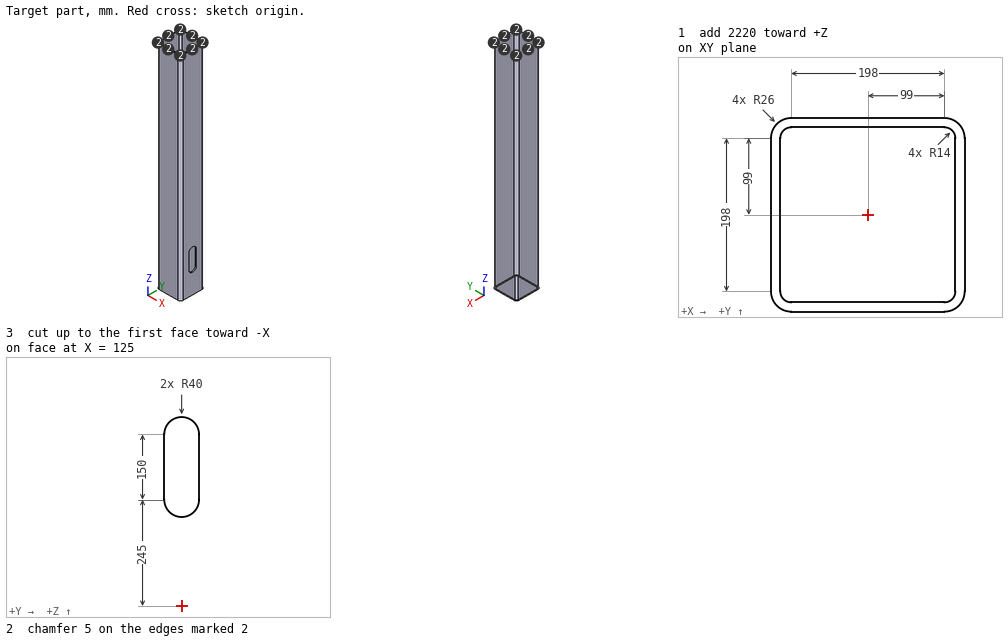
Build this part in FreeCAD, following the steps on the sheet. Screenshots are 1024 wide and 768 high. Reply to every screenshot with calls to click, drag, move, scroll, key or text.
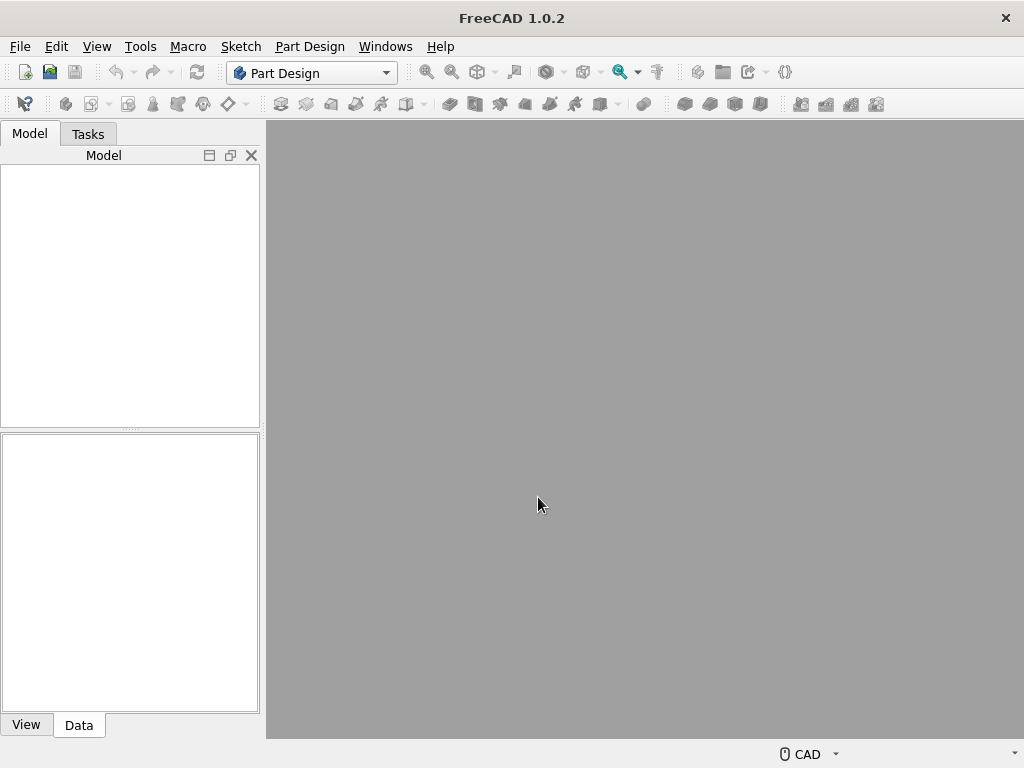
click(25, 72)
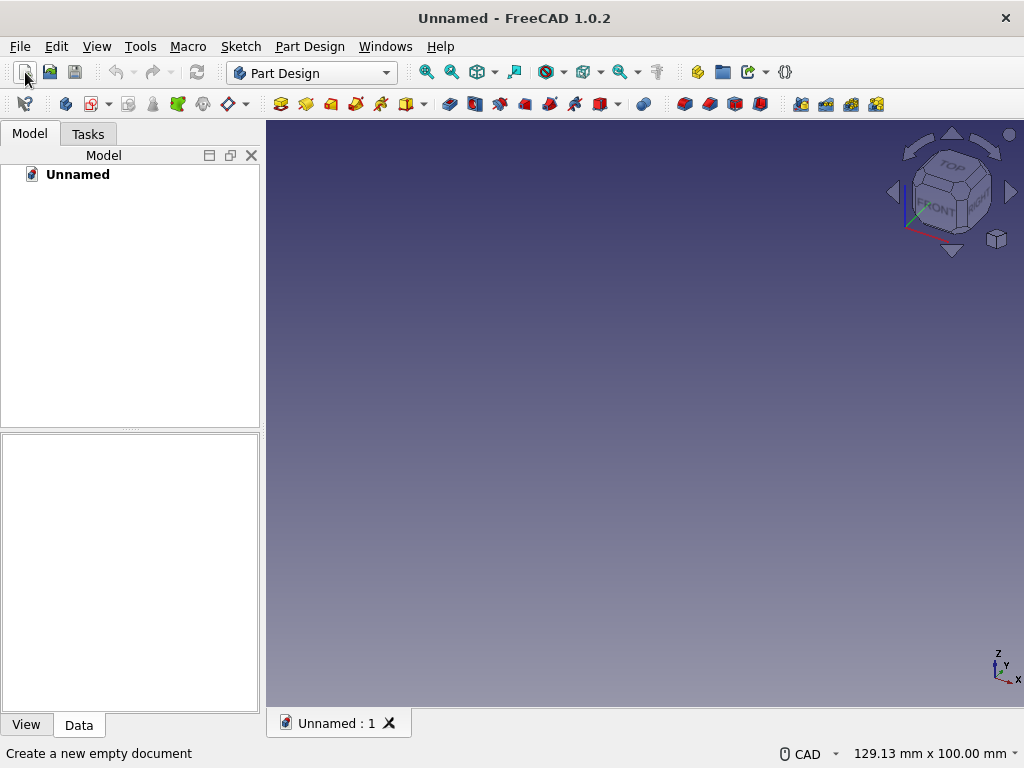
click(90, 104)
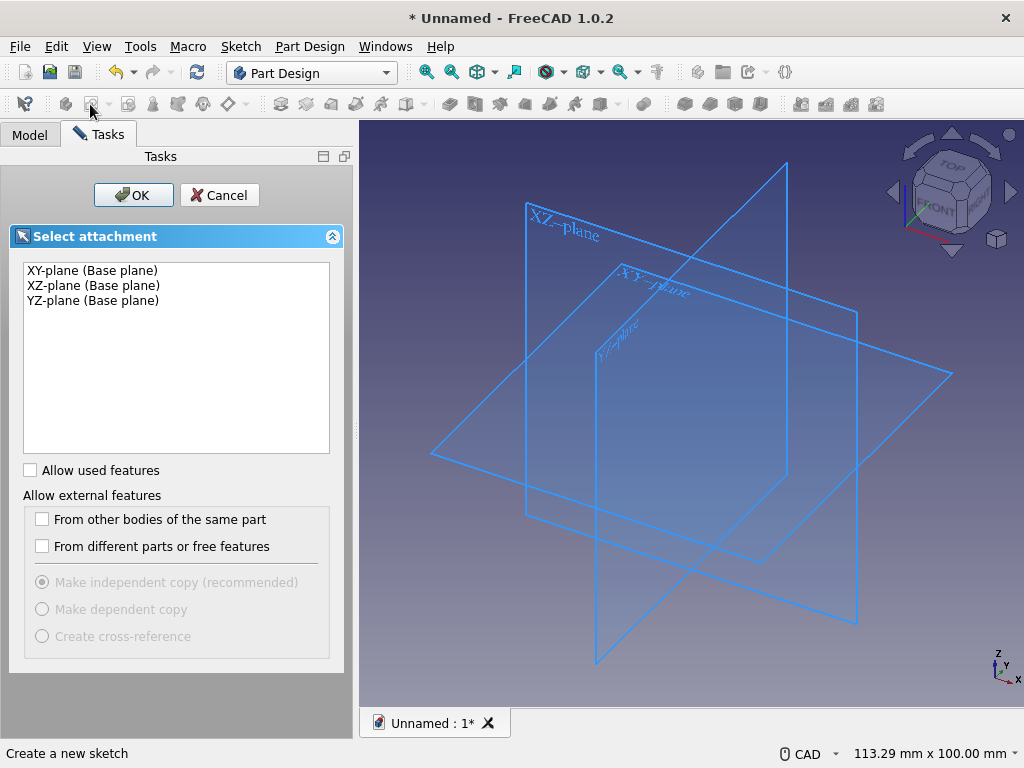
click(84, 270)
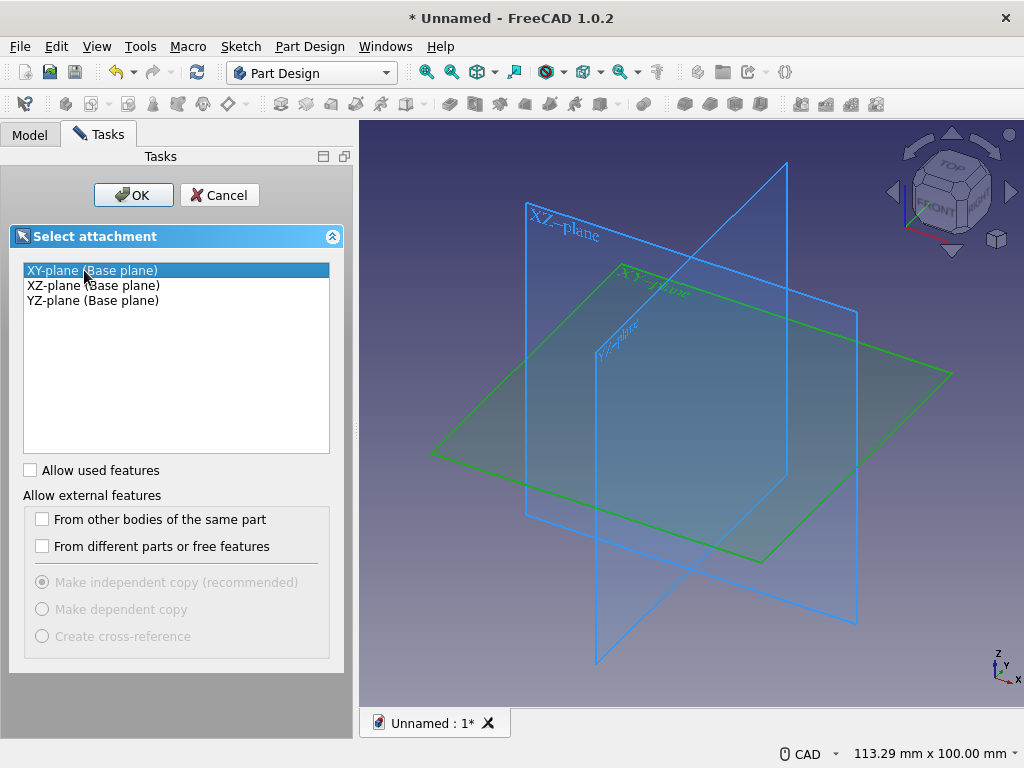
click(134, 195)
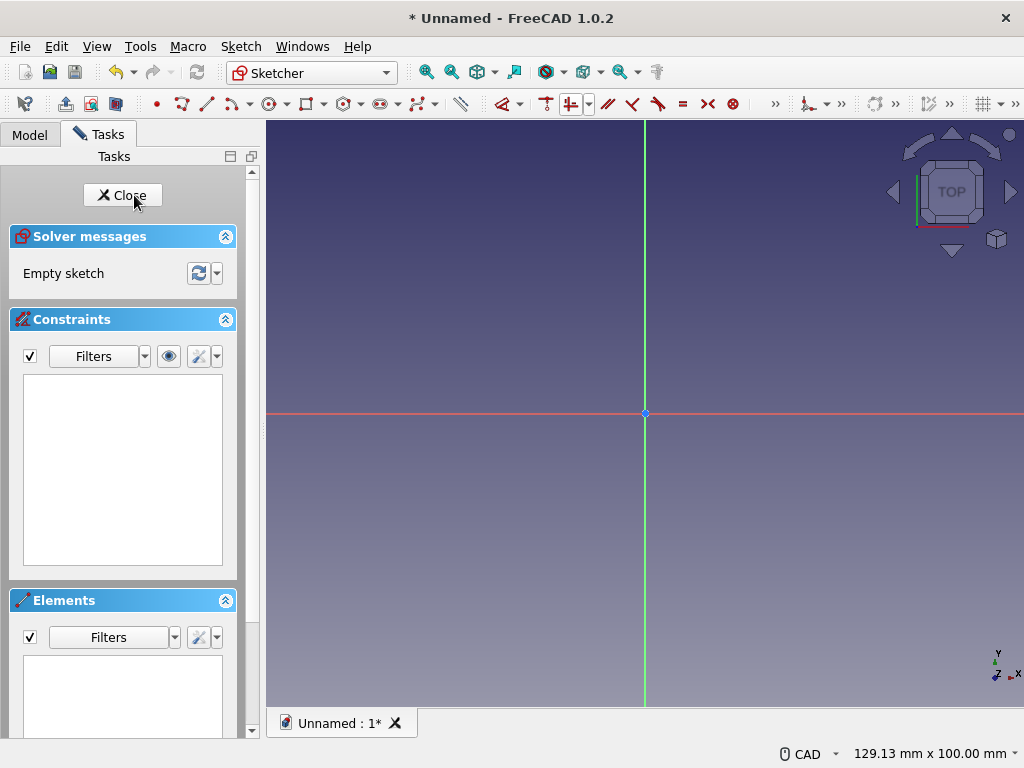
scroll(554, 414, down, 7)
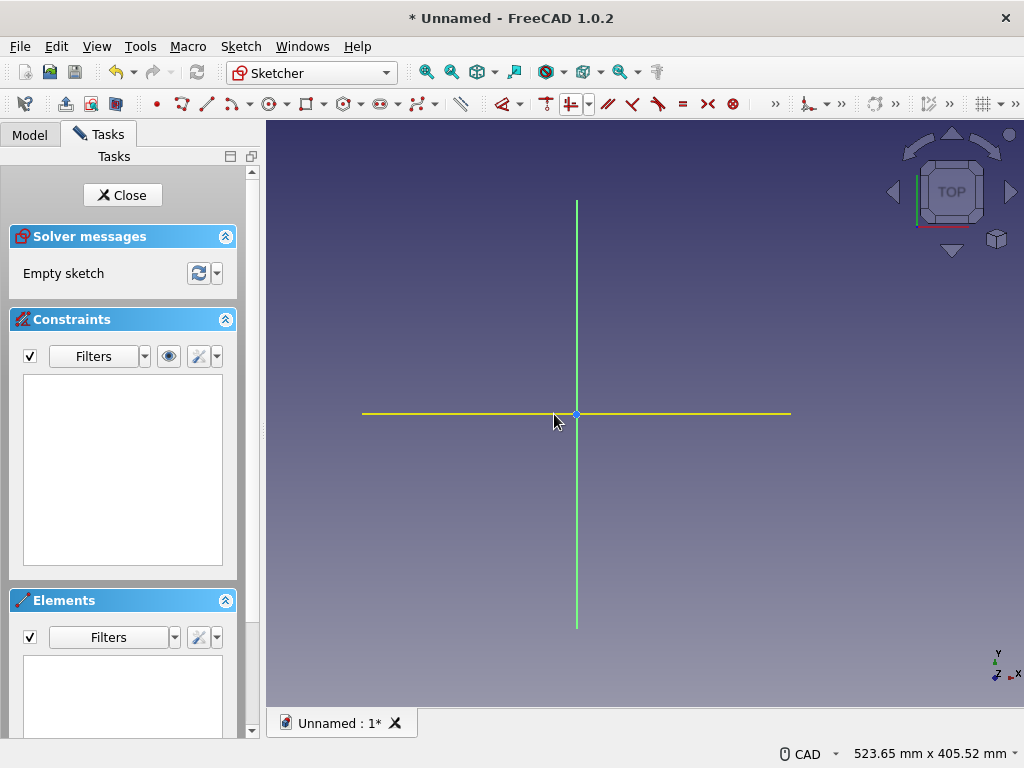
click(207, 104)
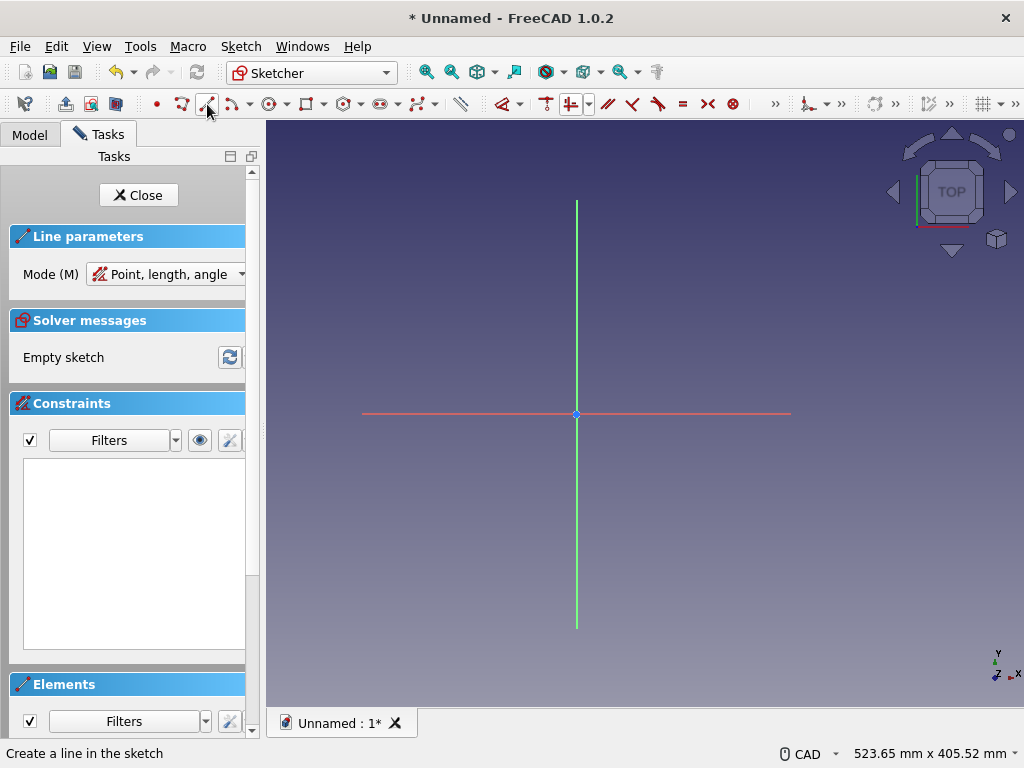
click(720, 233)
click(433, 233)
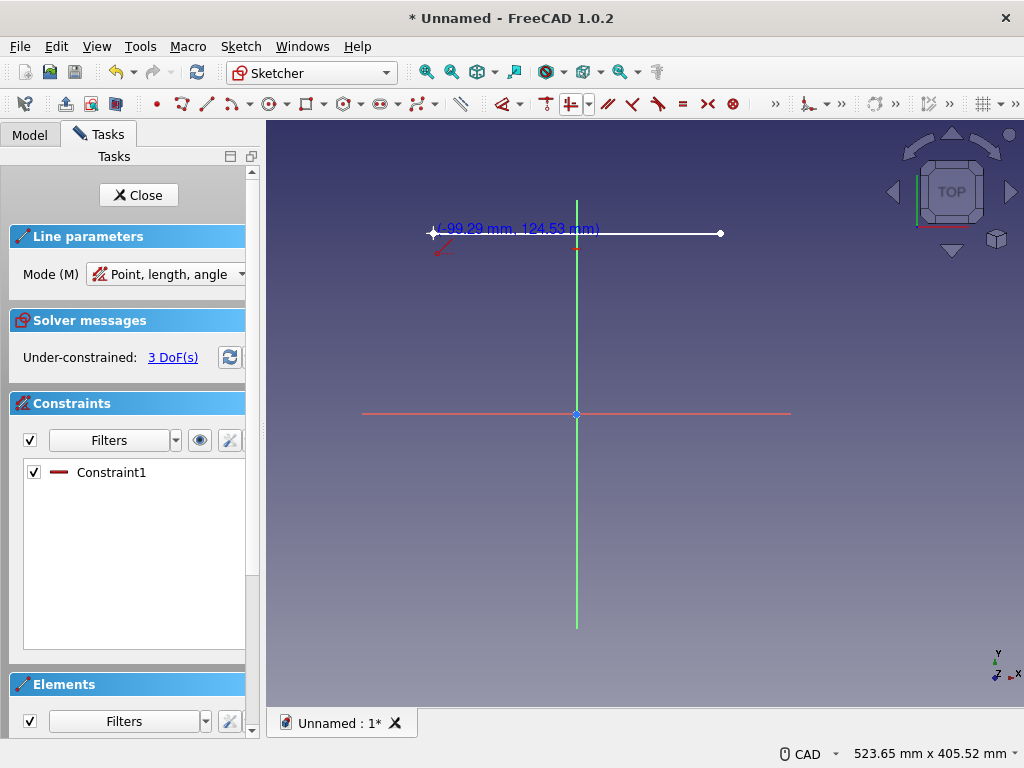
click(396, 271)
click(396, 558)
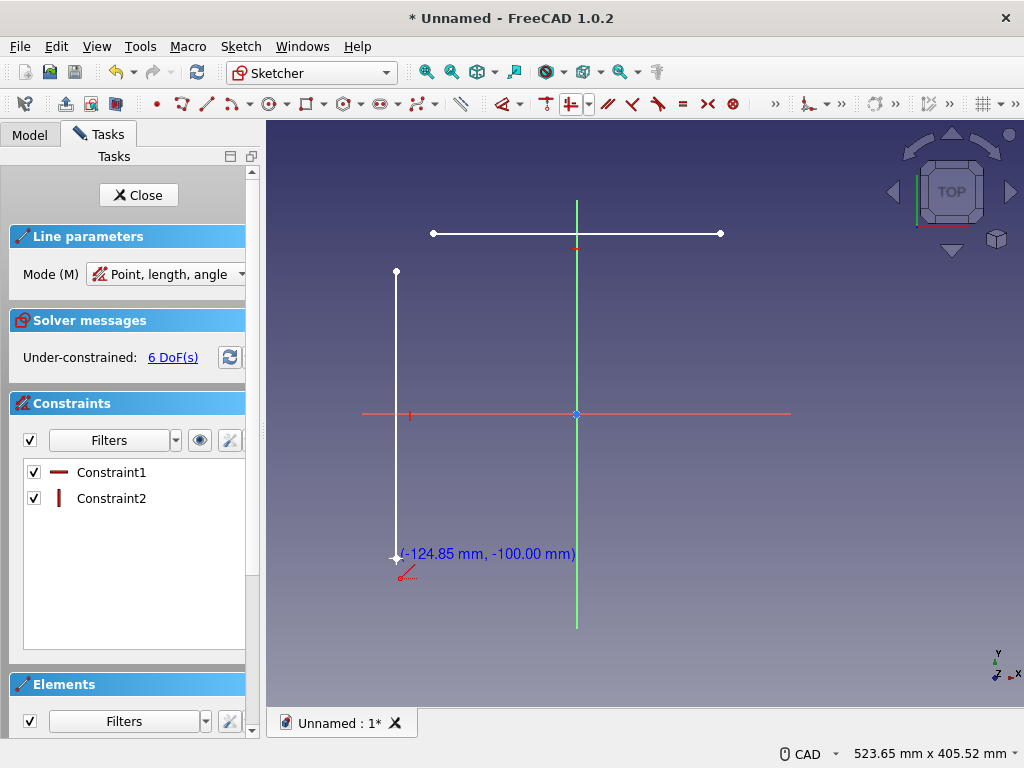
click(433, 595)
click(720, 595)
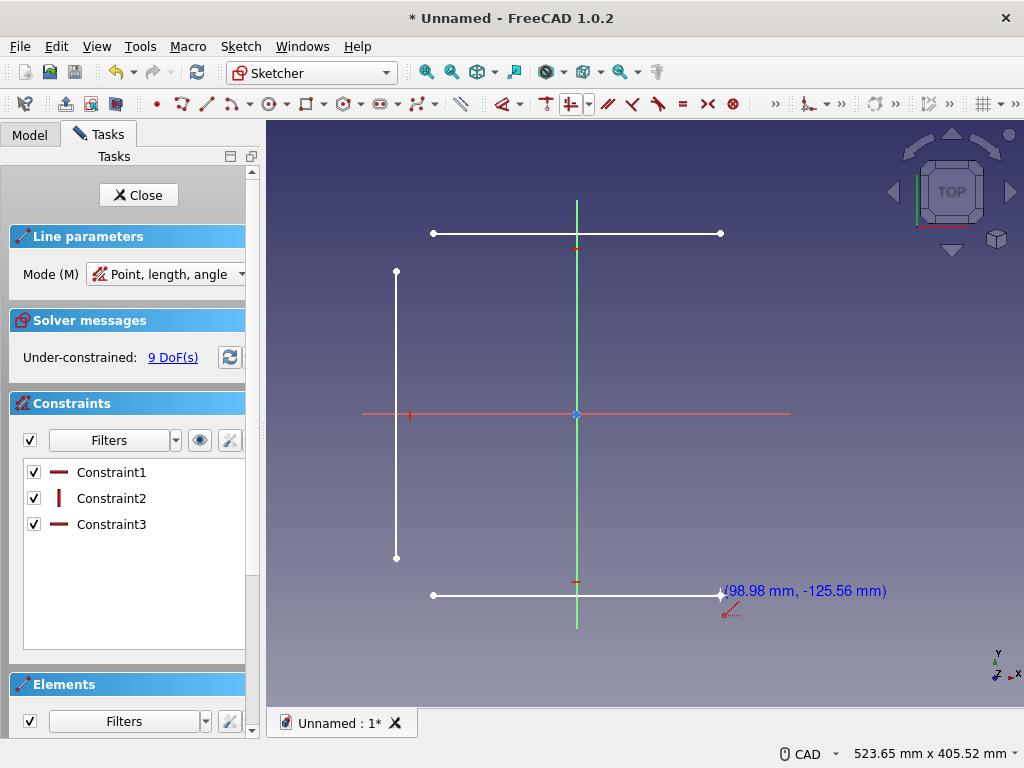
click(758, 558)
click(758, 271)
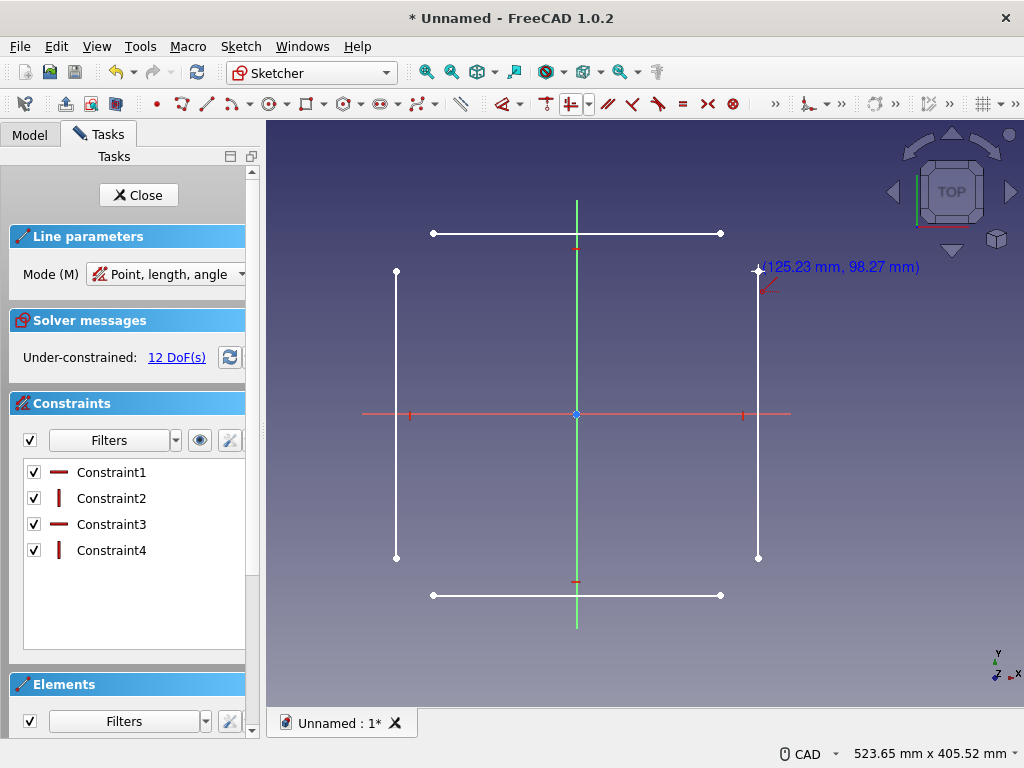
click(250, 104)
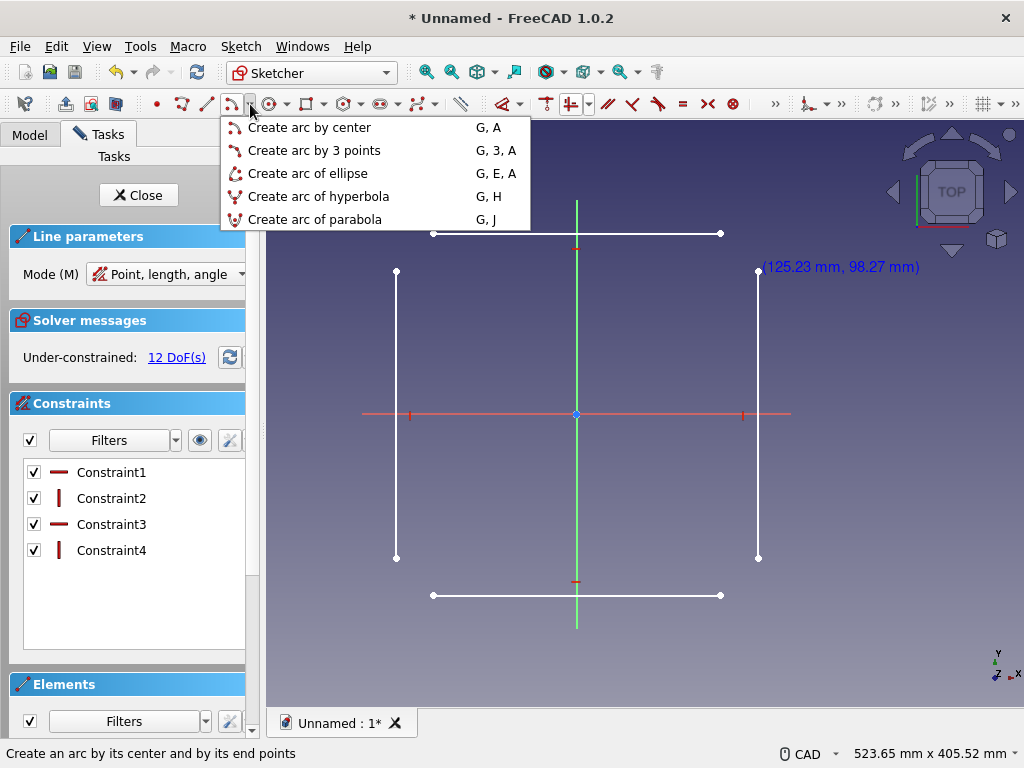
click(376, 150)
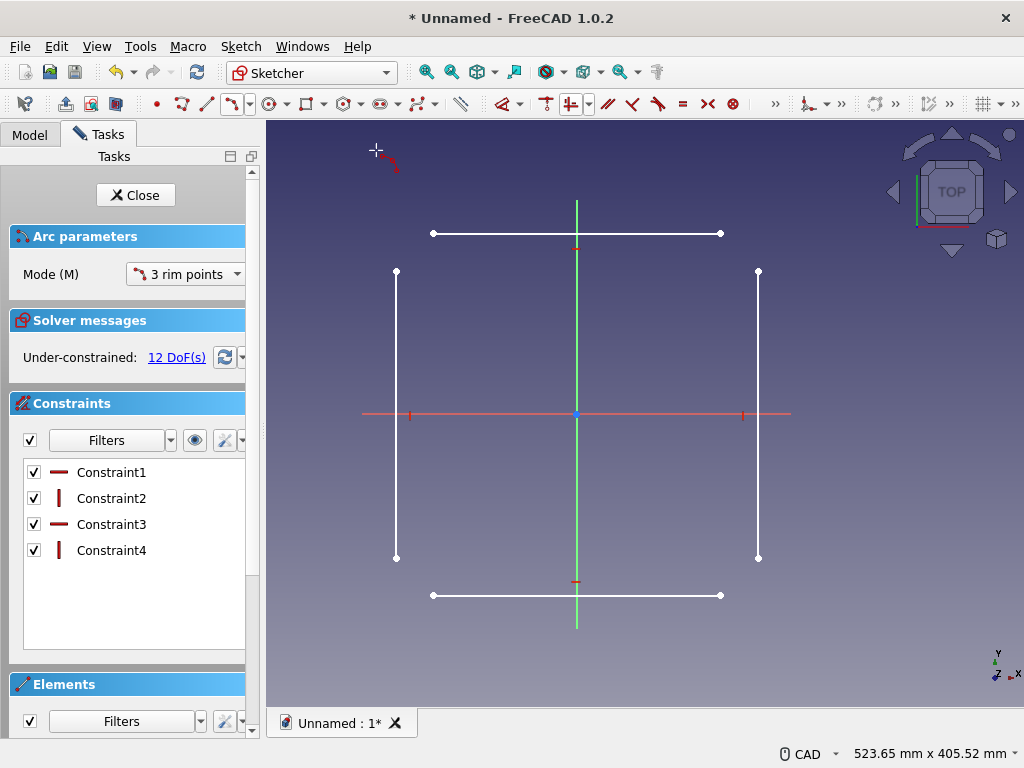
click(433, 234)
click(396, 272)